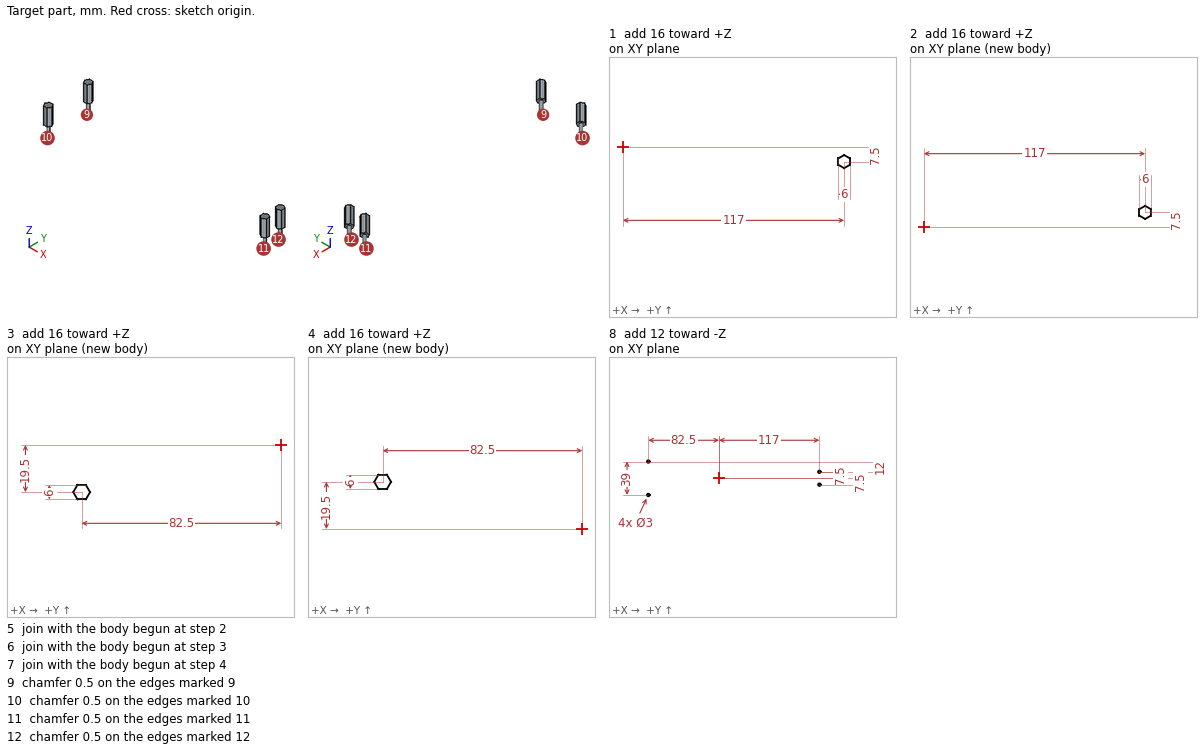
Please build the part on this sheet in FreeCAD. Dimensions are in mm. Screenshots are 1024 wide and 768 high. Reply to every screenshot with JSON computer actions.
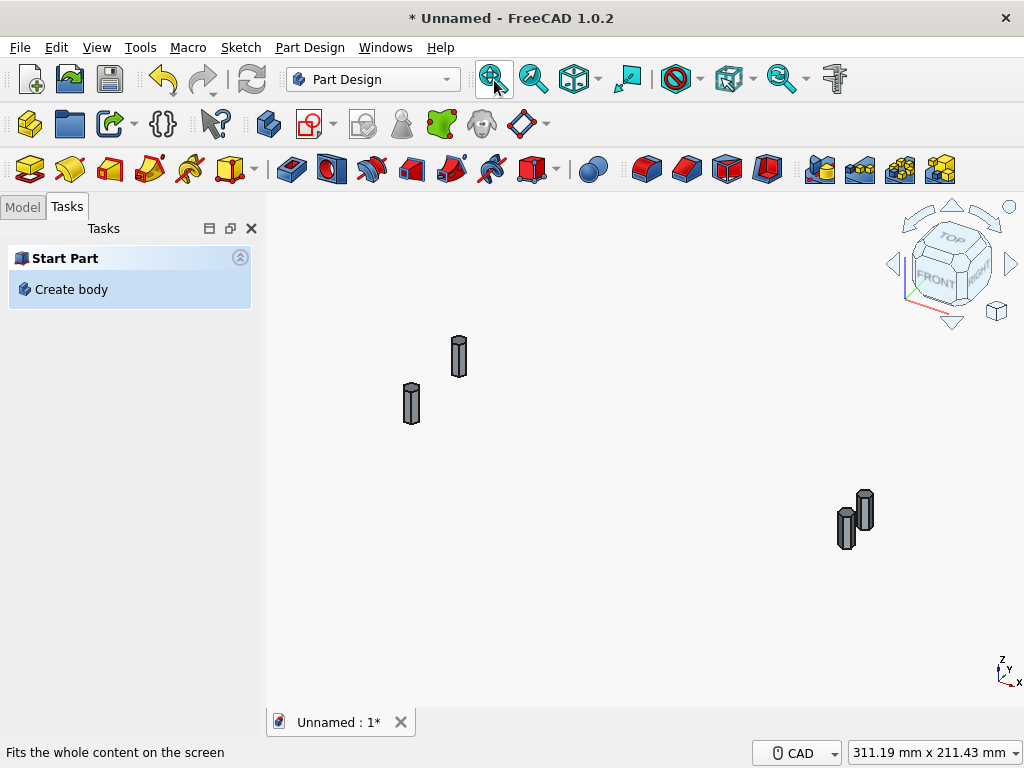
{"action": "left_click", "coordinate": [23, 206]}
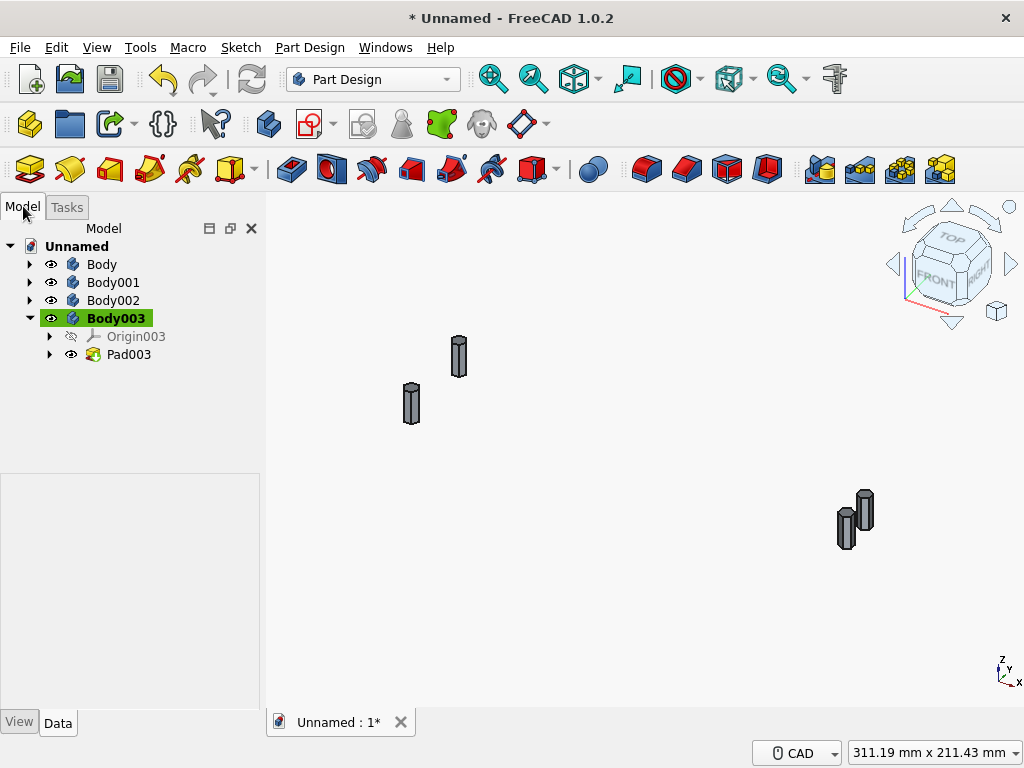
{"action": "double_click", "coordinate": [96, 264]}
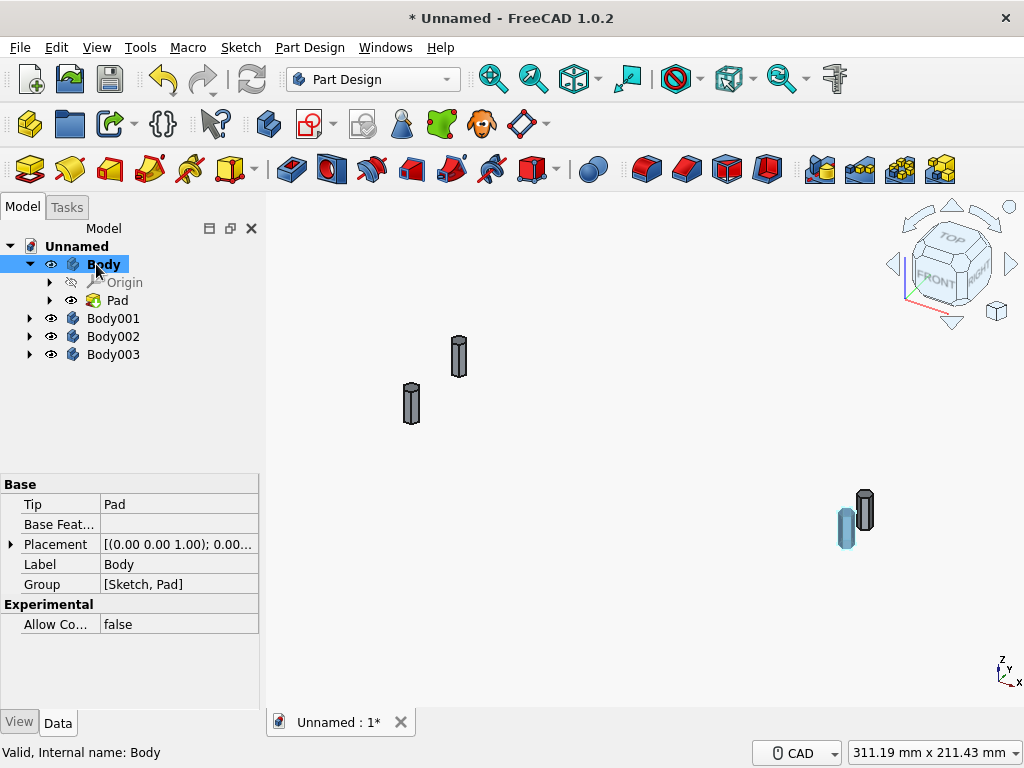
{"action": "left_click", "coordinate": [96, 264]}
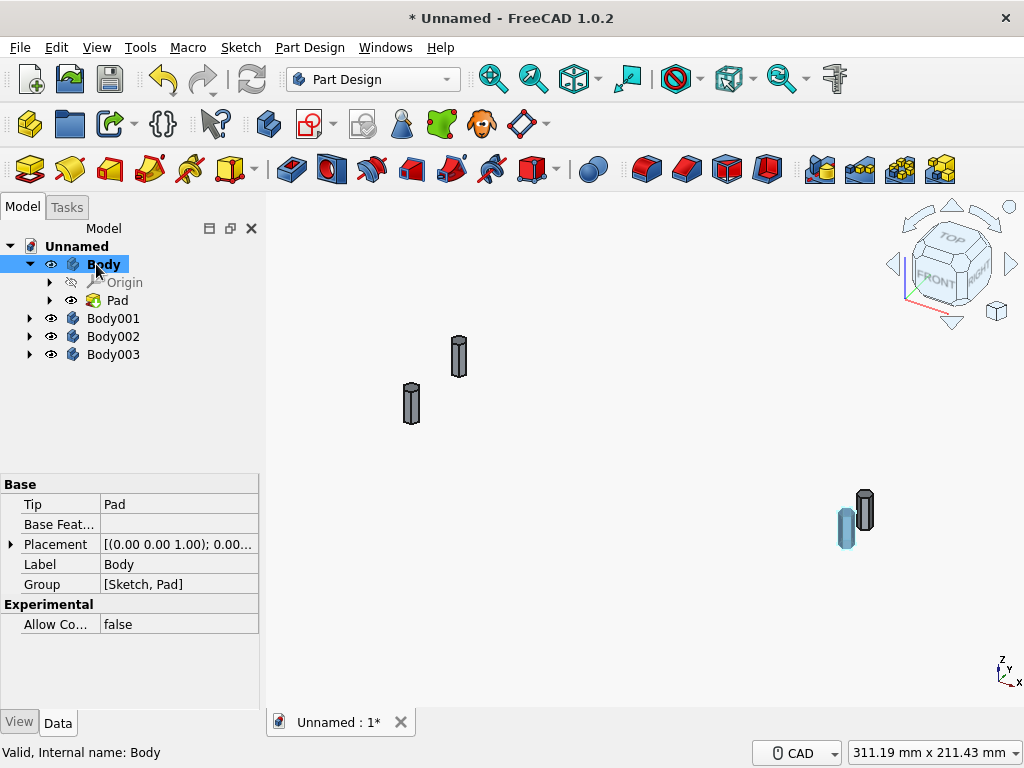
{"action": "left_click", "coordinate": [146, 624]}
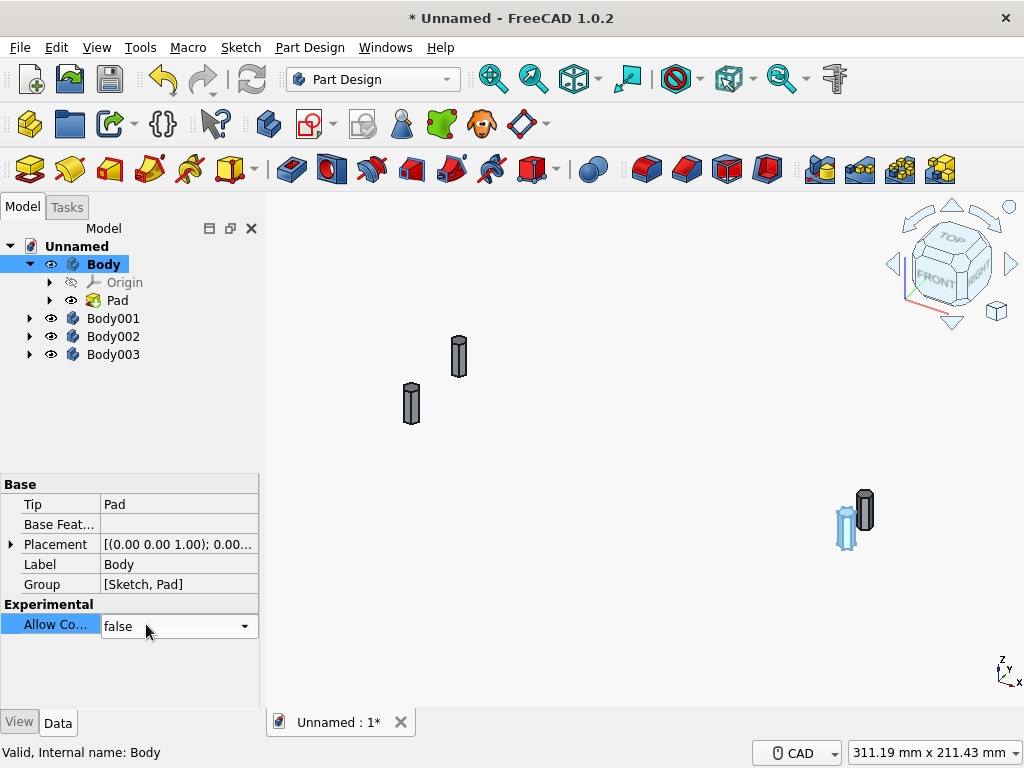
{"action": "left_click", "coordinate": [146, 624]}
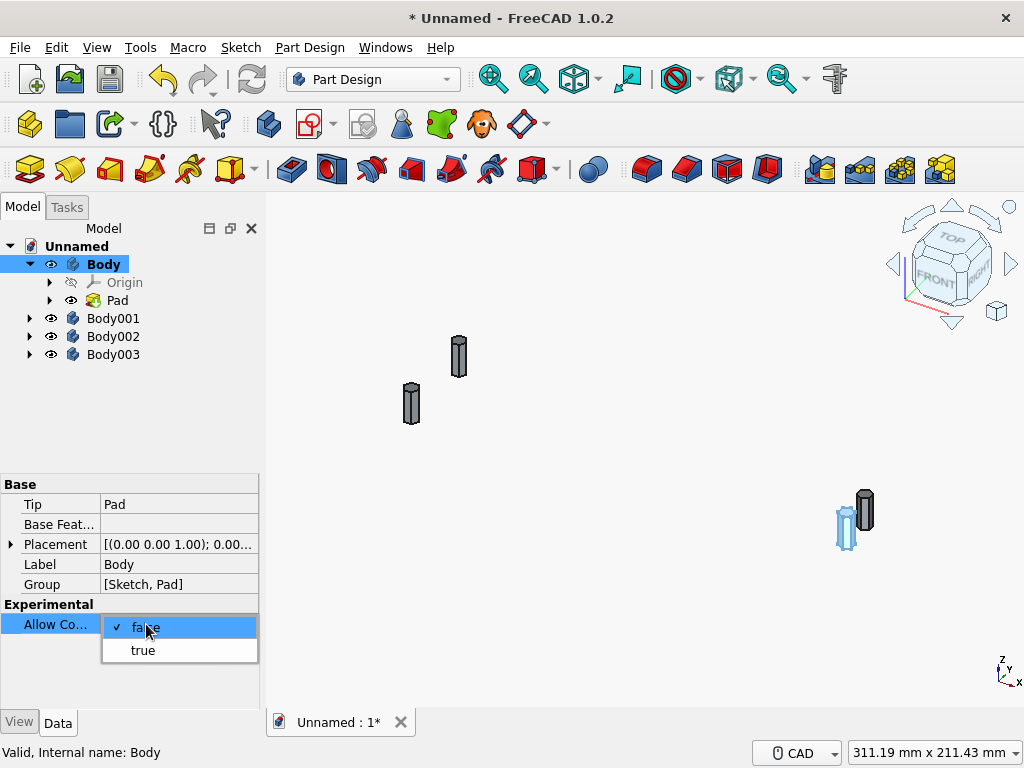
{"action": "left_click", "coordinate": [179, 650]}
{"action": "key", "text": "Return"}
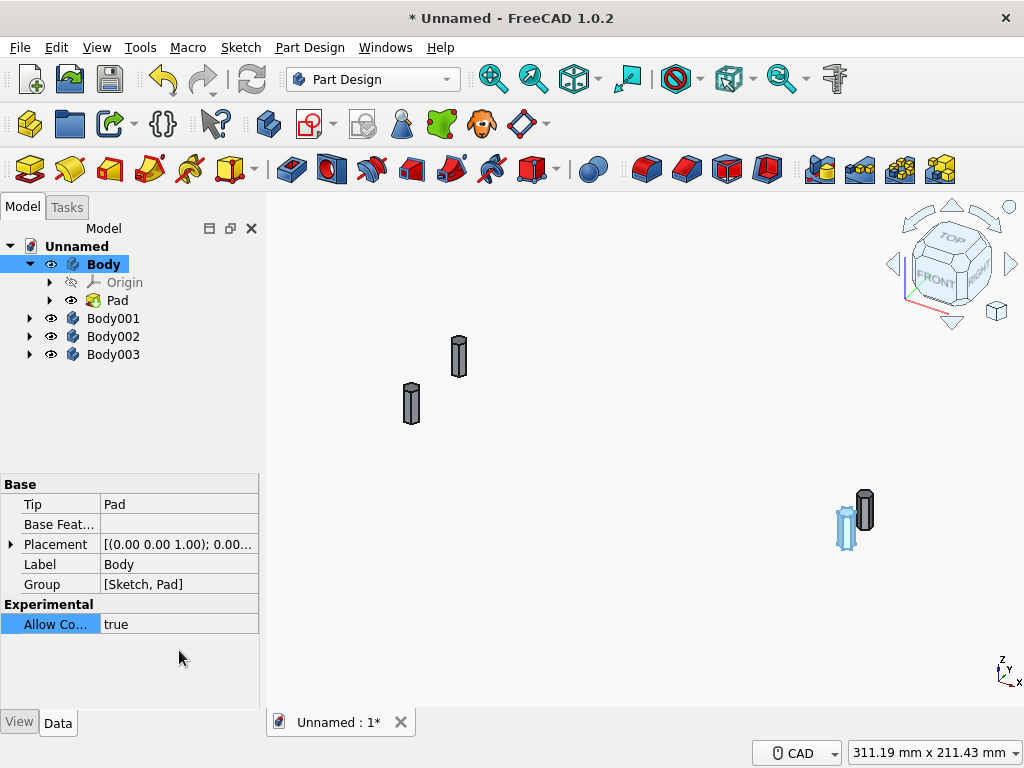
{"action": "left_click", "coordinate": [96, 318]}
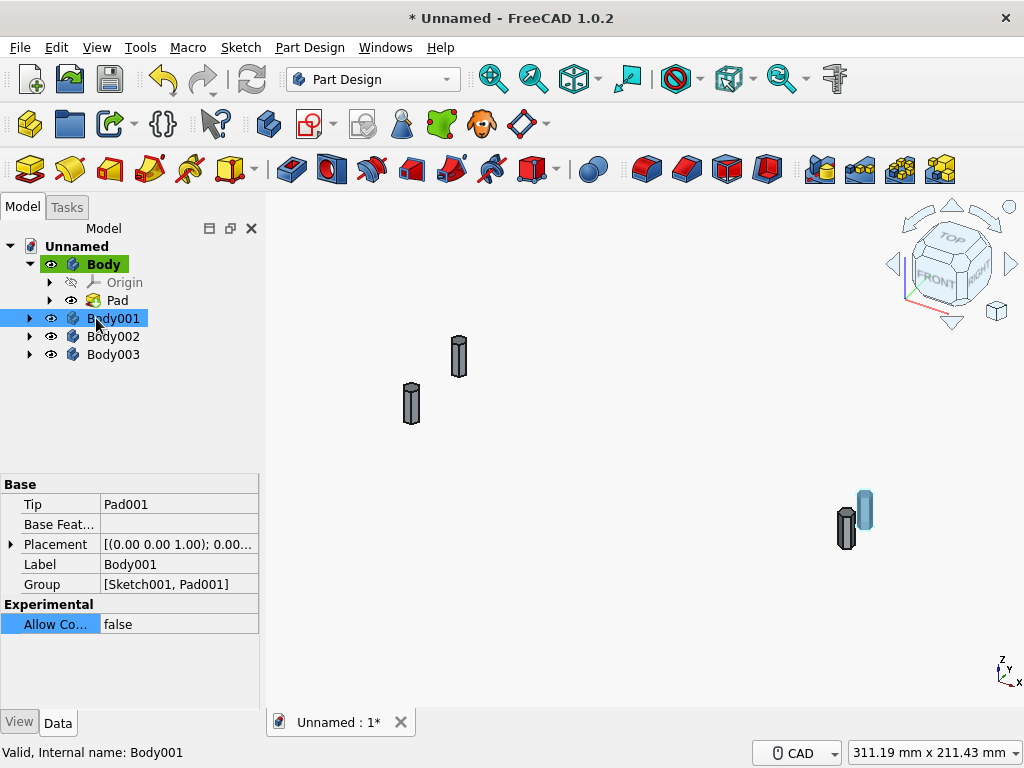
{"action": "left_click", "coordinate": [594, 170]}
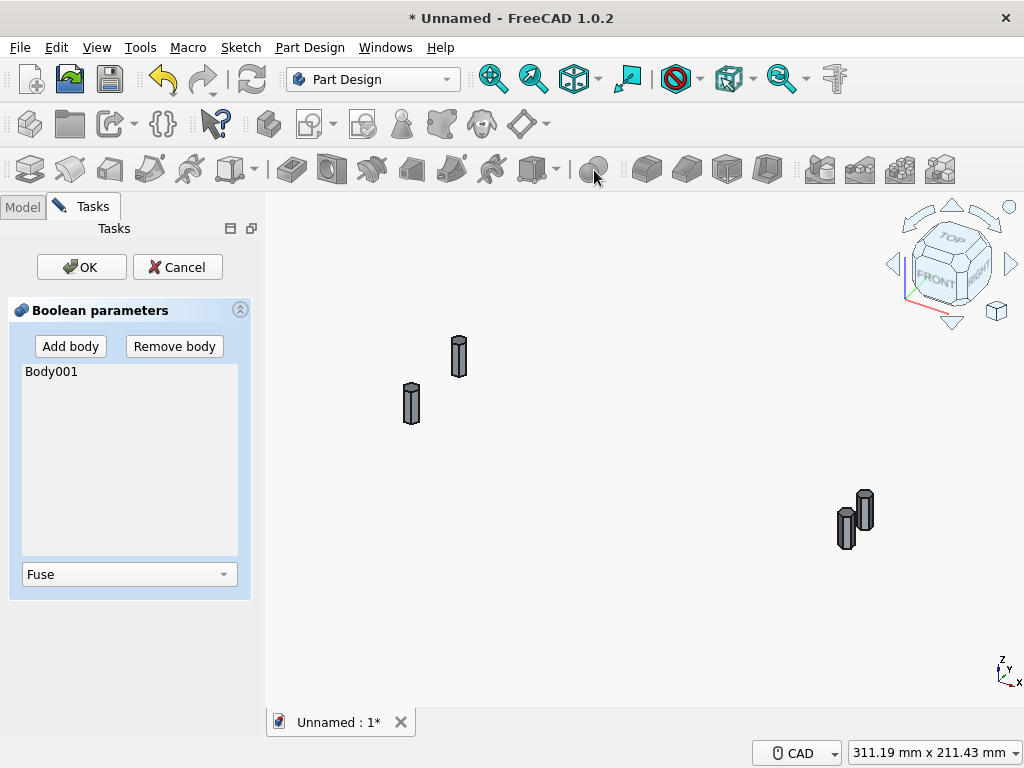
{"action": "left_click", "coordinate": [82, 267]}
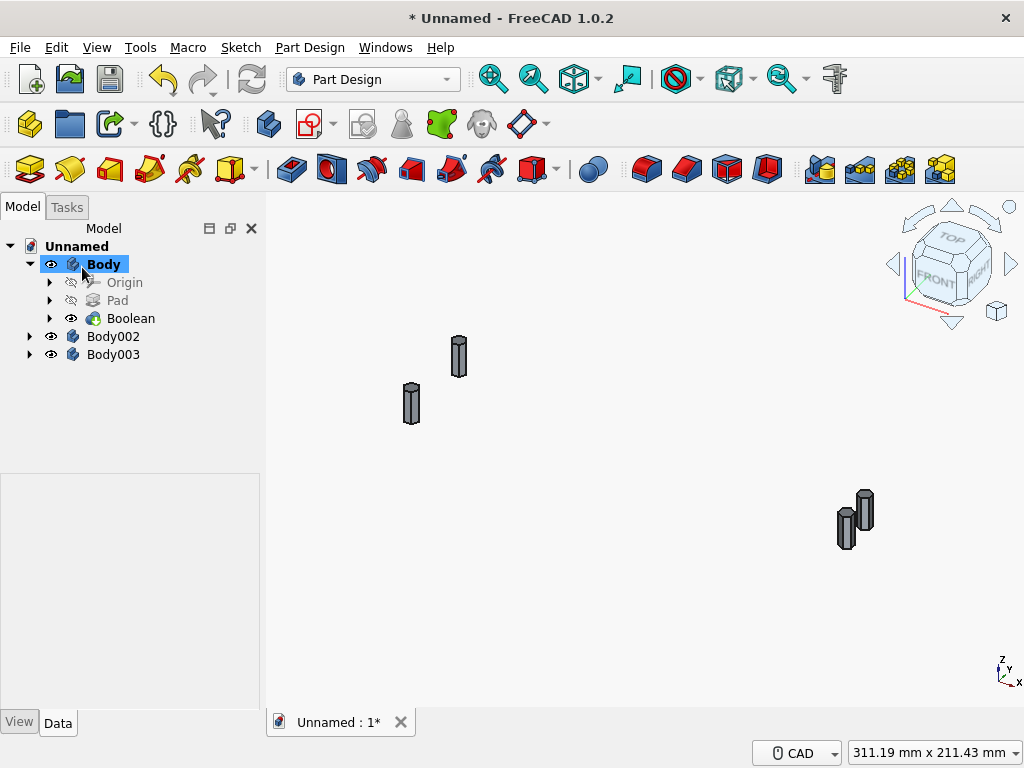
{"action": "left_click", "coordinate": [494, 80]}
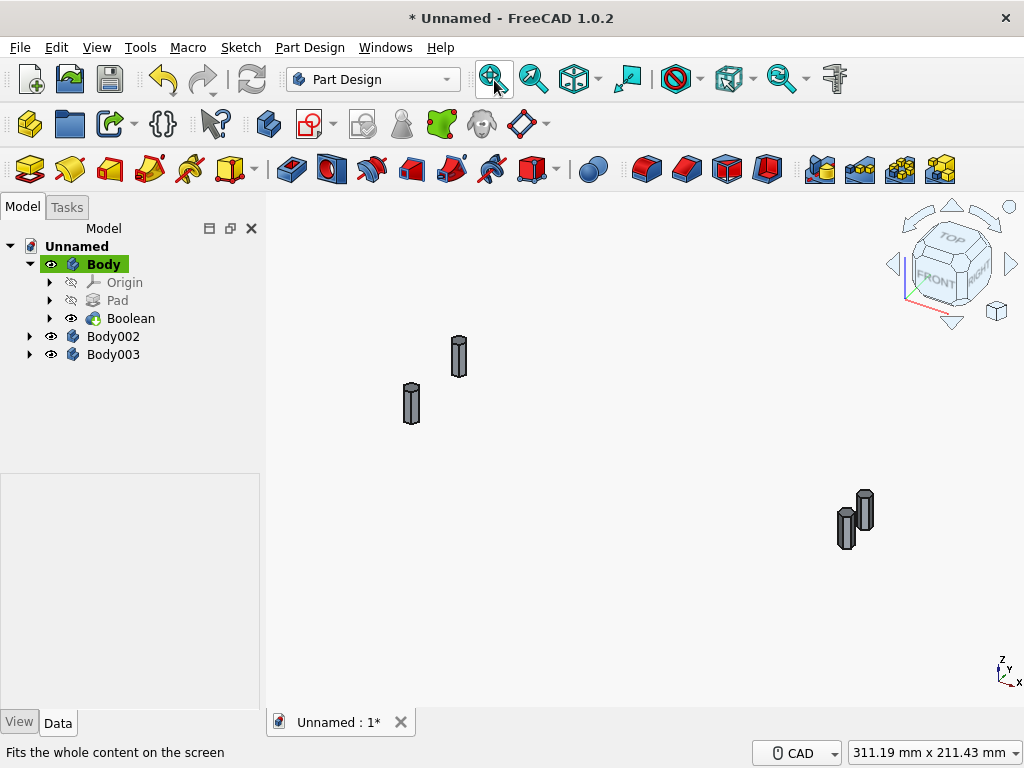
{"action": "left_click", "coordinate": [96, 336]}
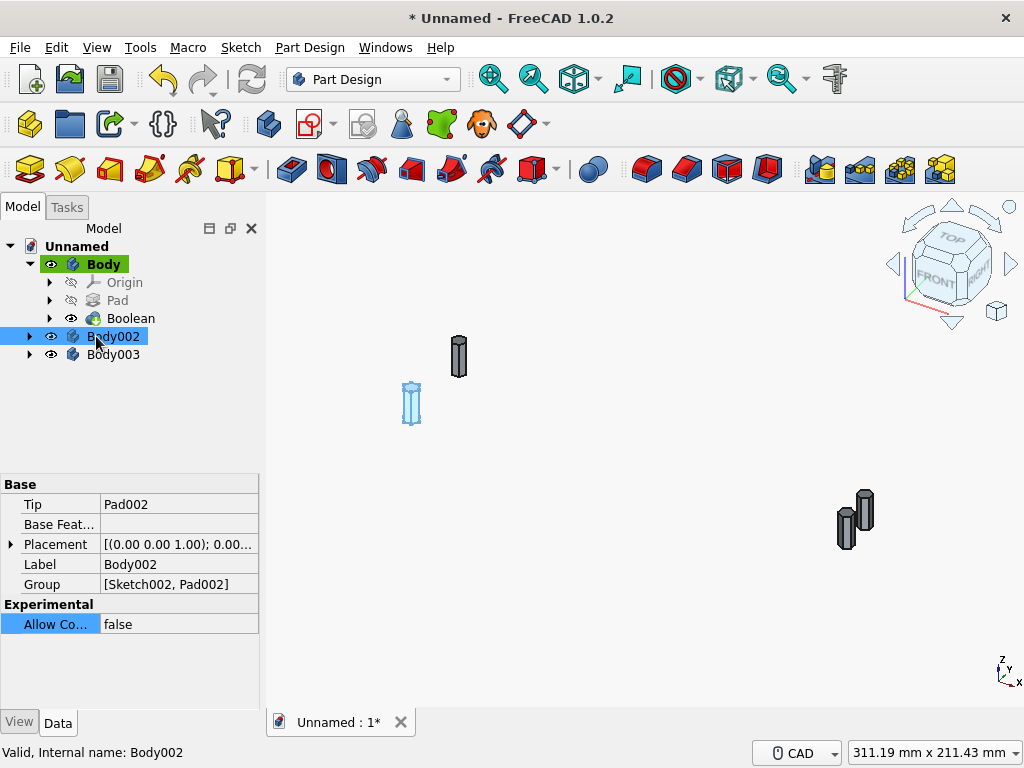
{"action": "left_click", "coordinate": [594, 170]}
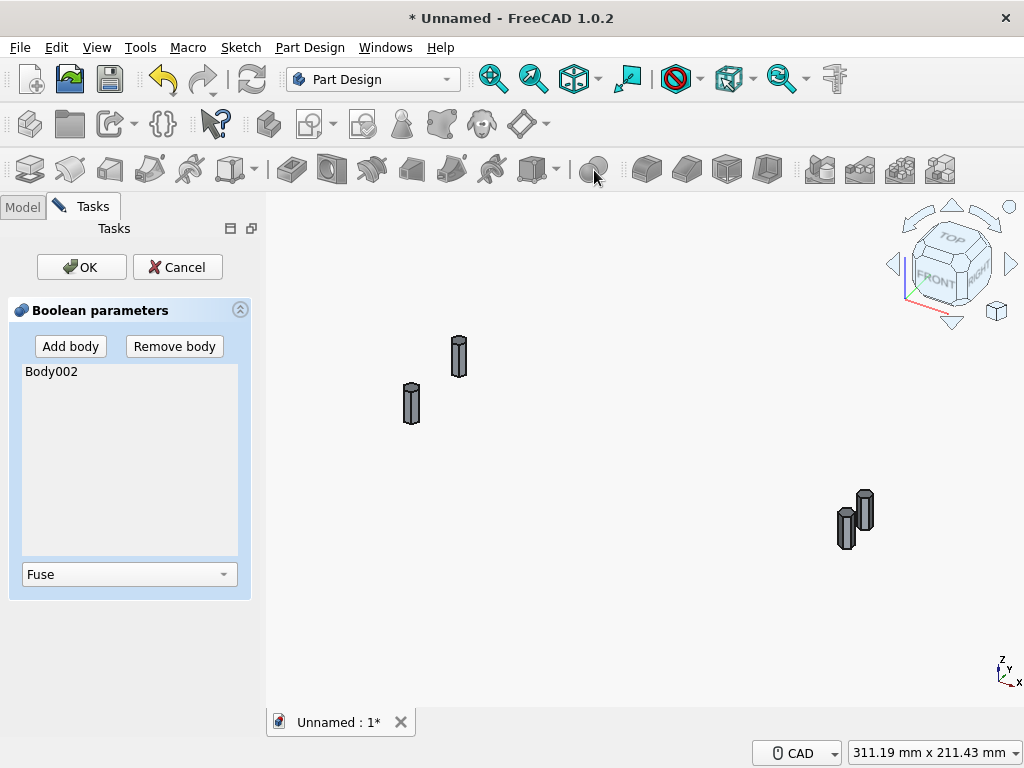
{"action": "left_click", "coordinate": [82, 267]}